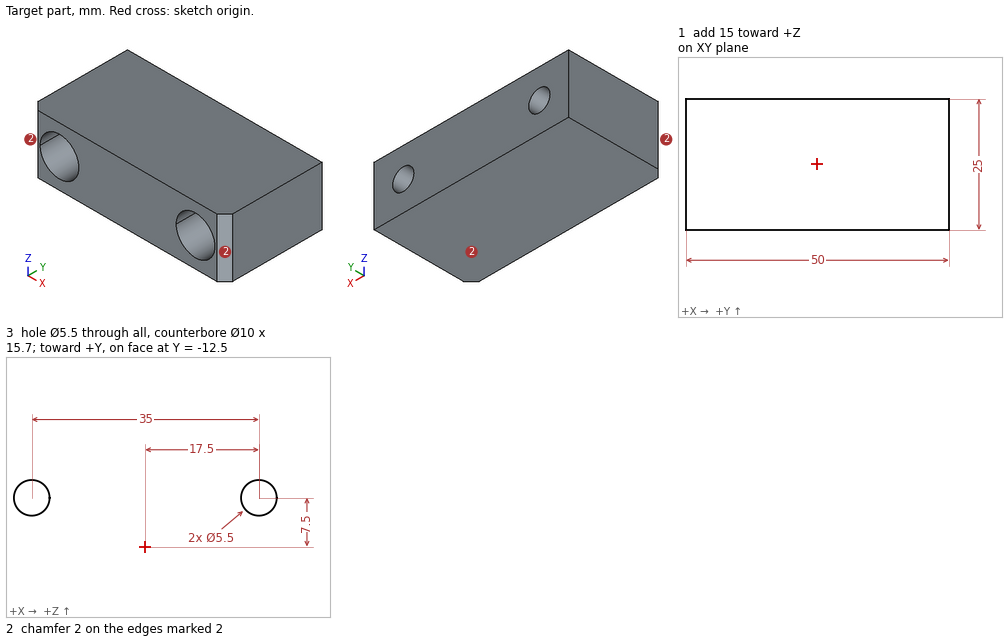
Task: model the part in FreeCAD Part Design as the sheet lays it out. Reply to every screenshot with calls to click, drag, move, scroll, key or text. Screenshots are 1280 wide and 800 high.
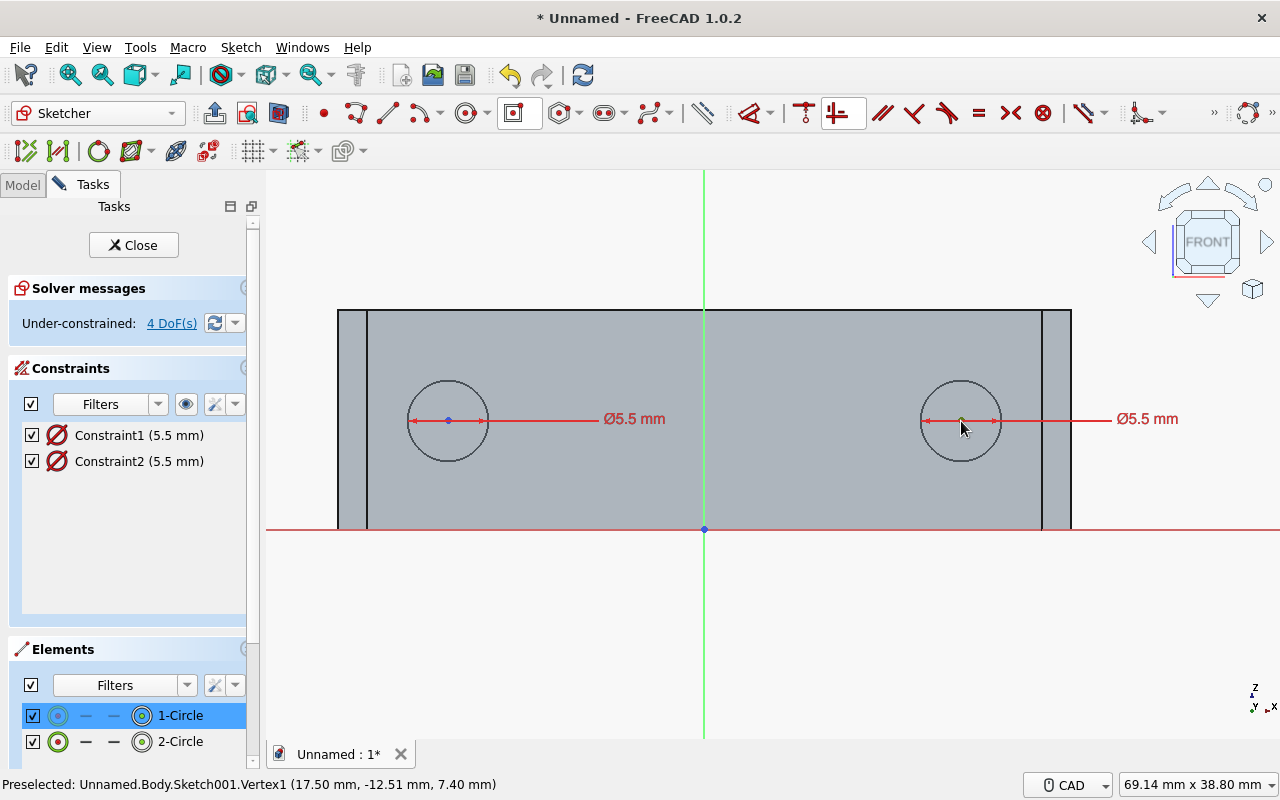
click(448, 421)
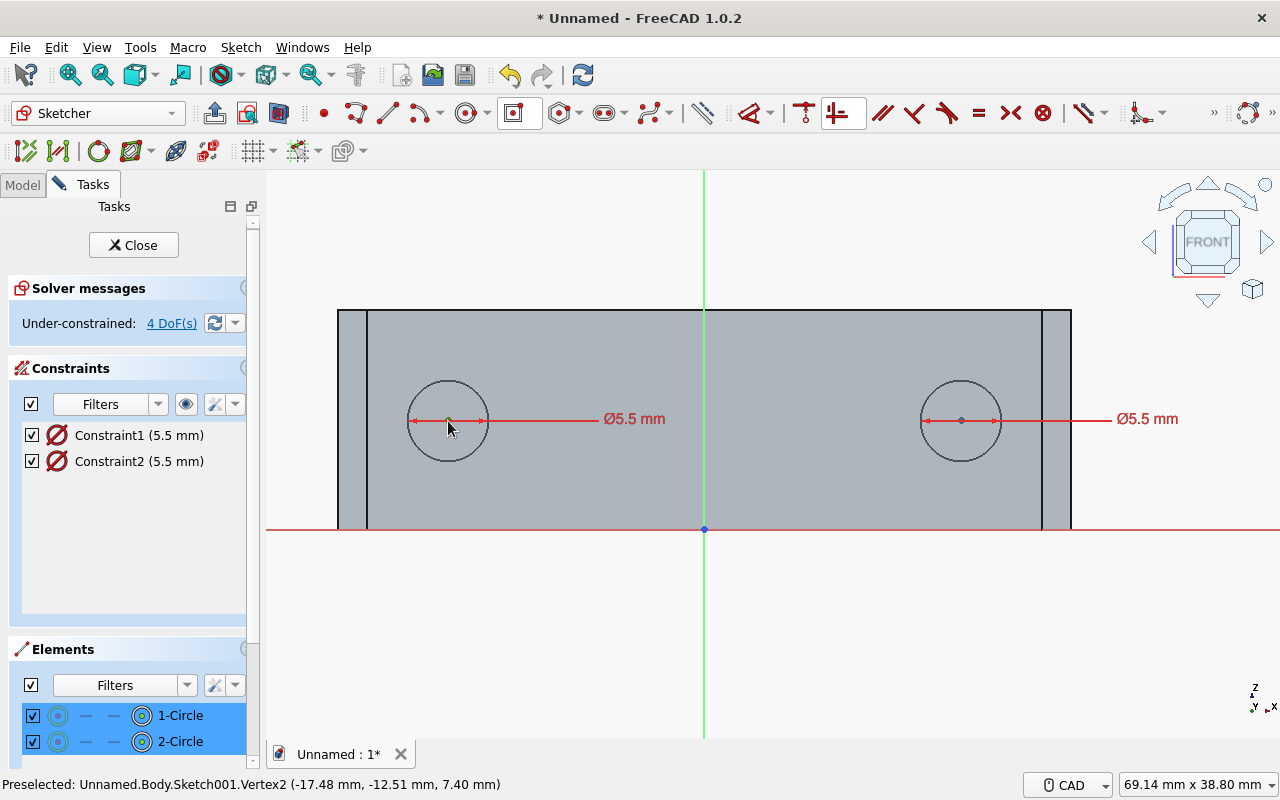
click(860, 114)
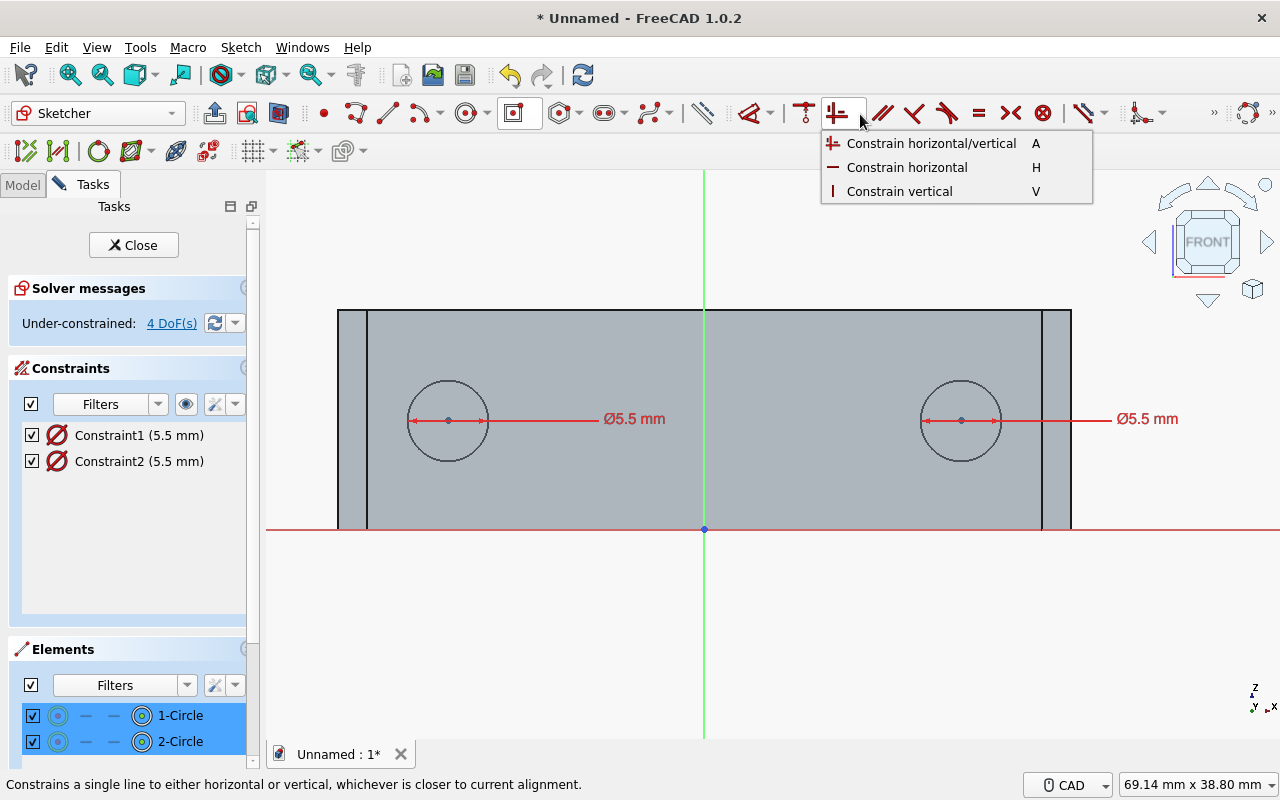
click(957, 167)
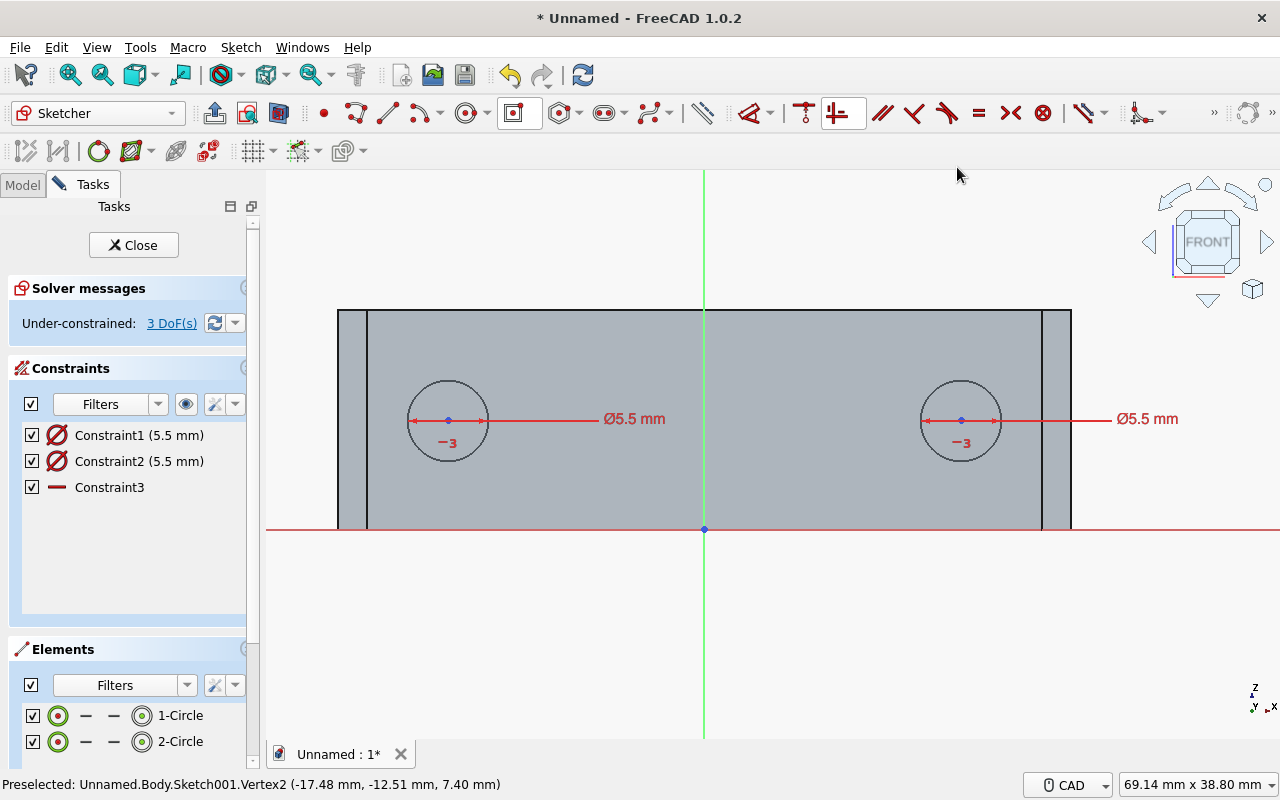
key(d)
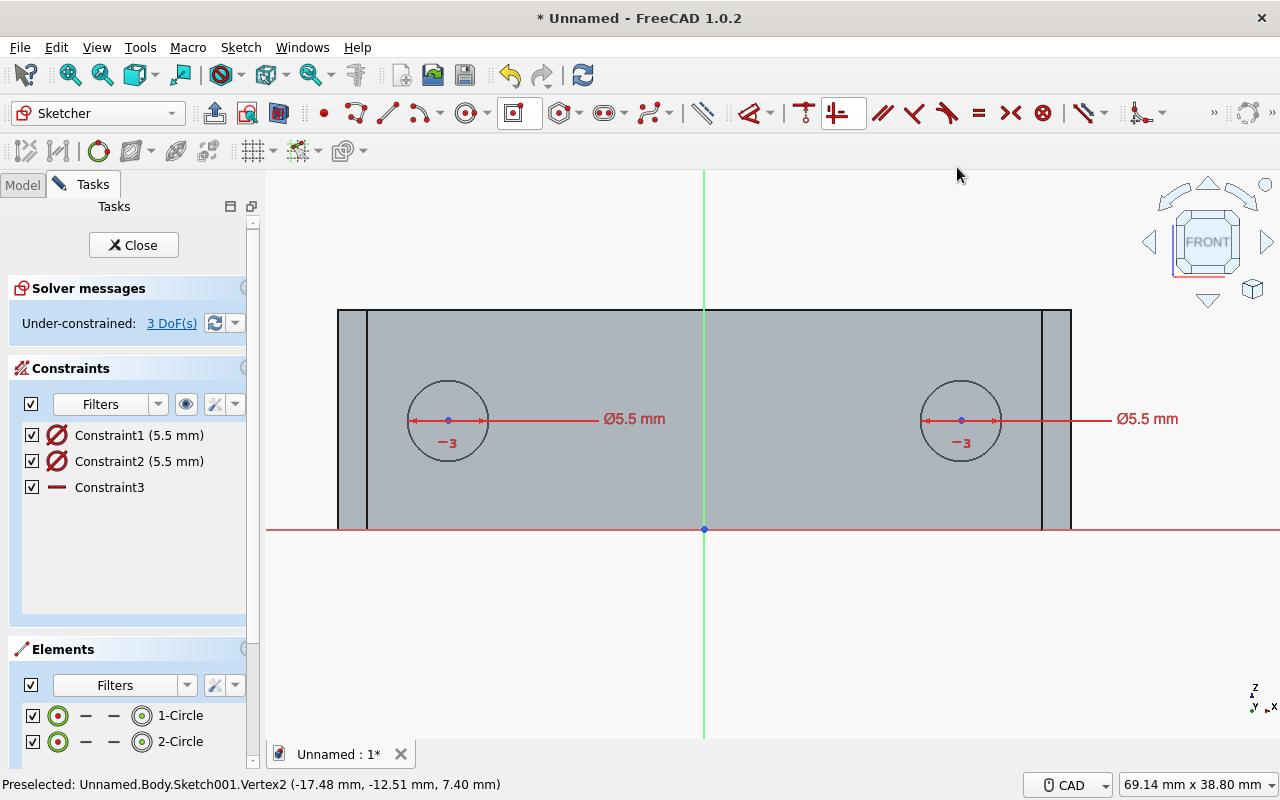
click(961, 421)
click(995, 475)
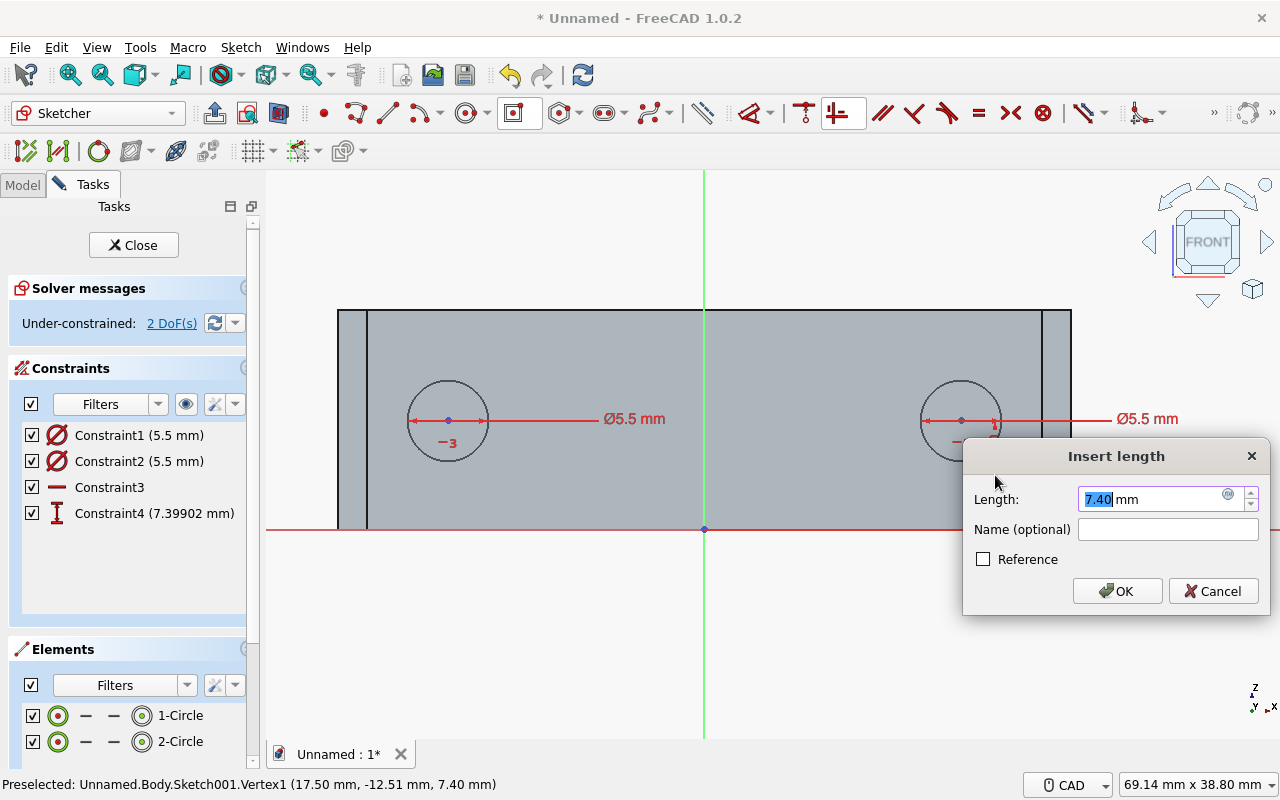
text(7.5)
key(Return)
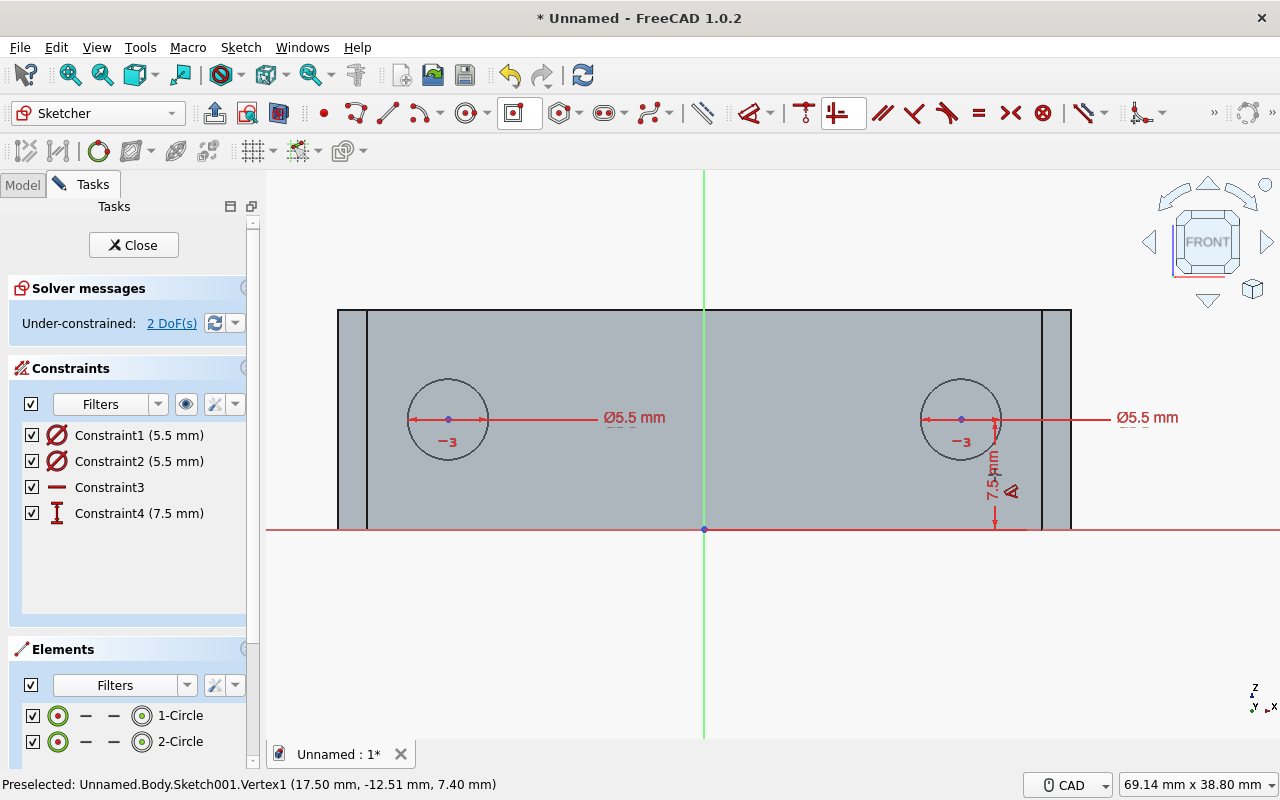
click(961, 420)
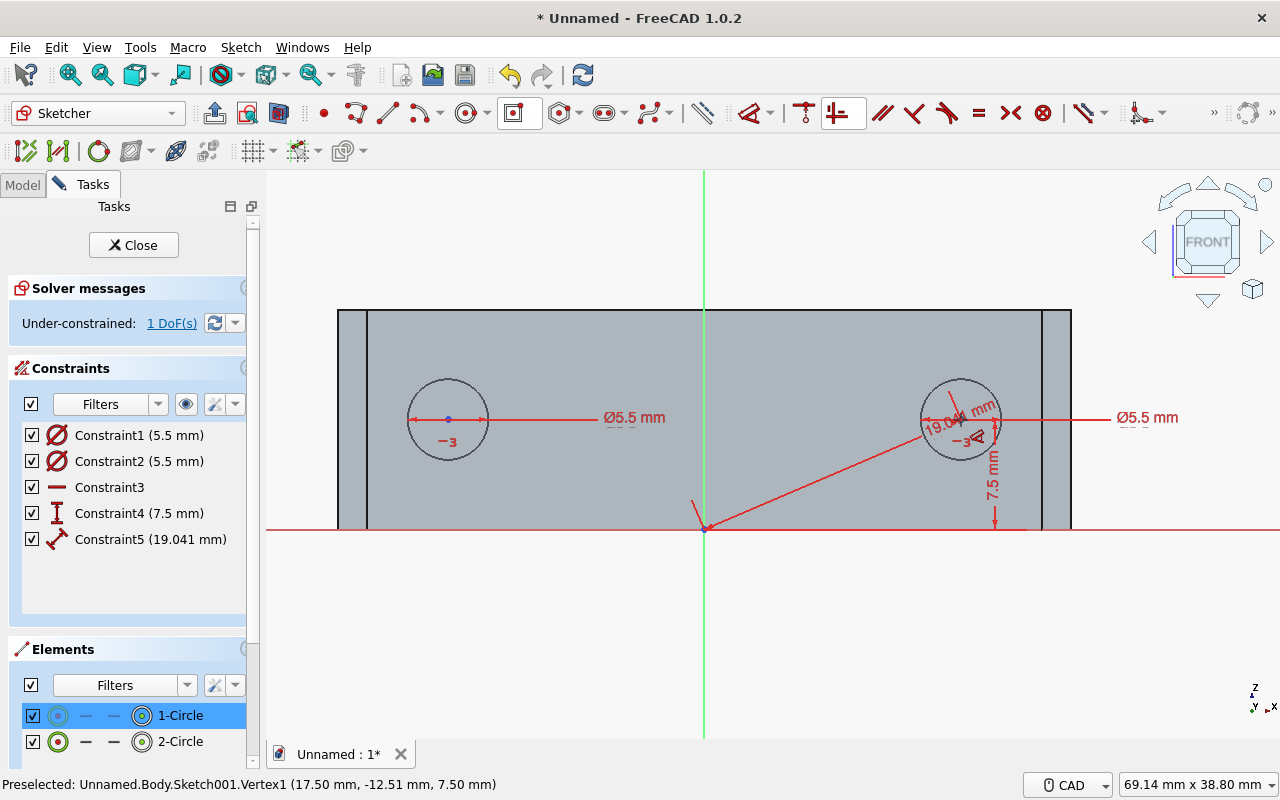
click(448, 420)
click(587, 386)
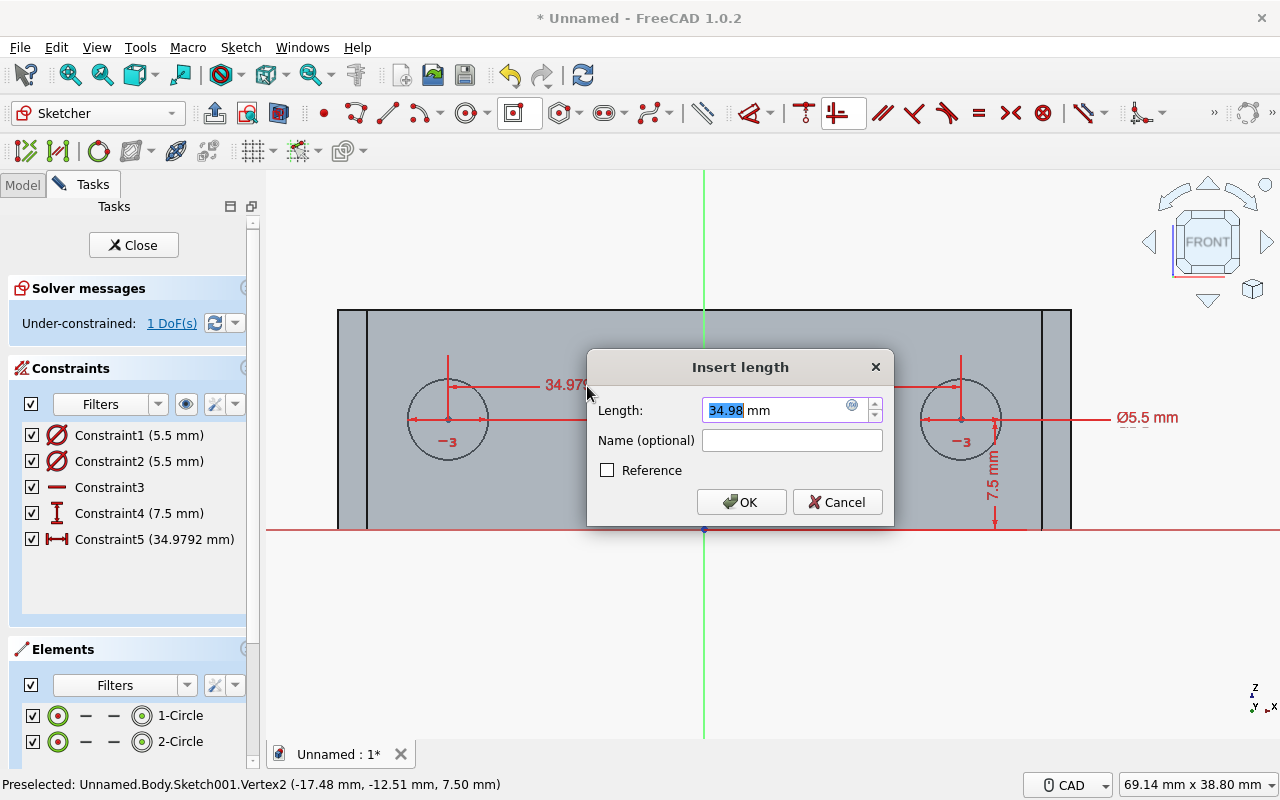
text(35)
key(Return)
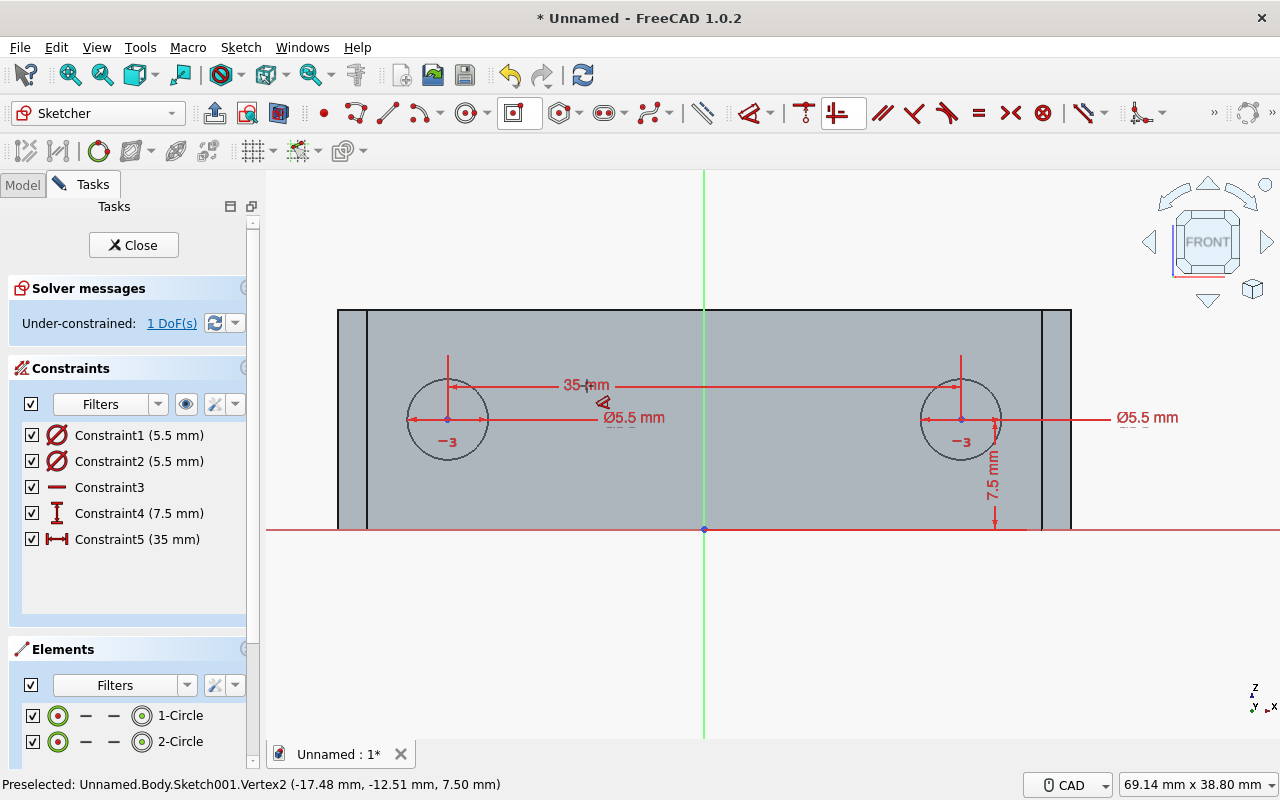
click(961, 420)
click(833, 564)